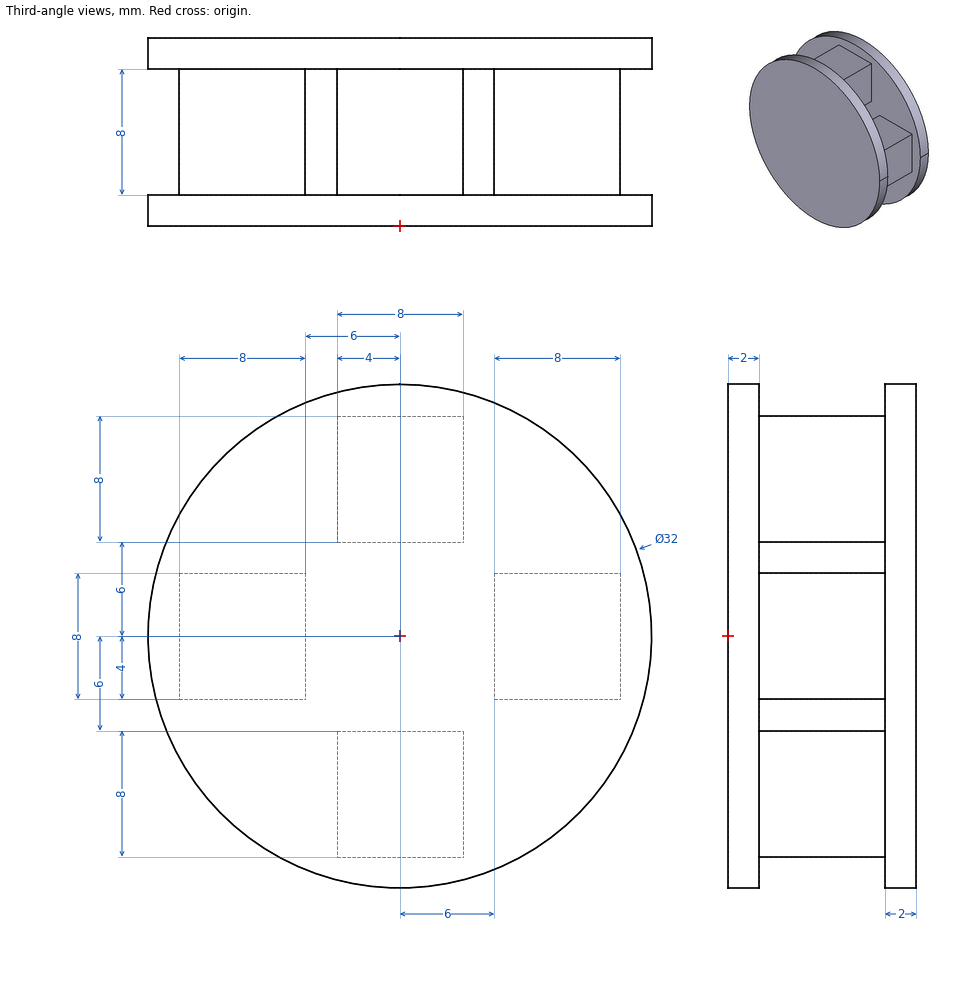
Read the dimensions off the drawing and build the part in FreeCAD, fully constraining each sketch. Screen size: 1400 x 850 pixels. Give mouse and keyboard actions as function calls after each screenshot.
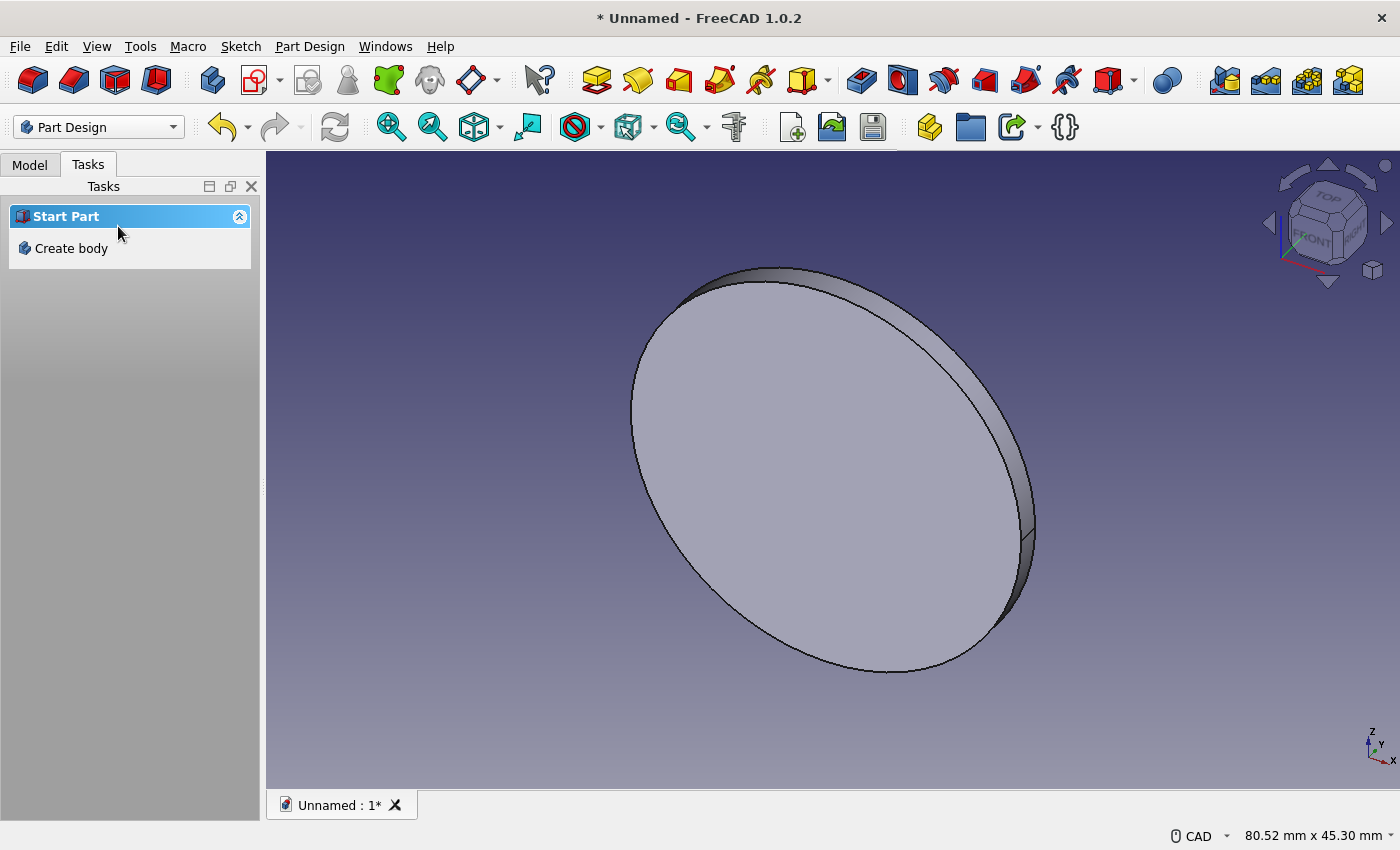
key(4)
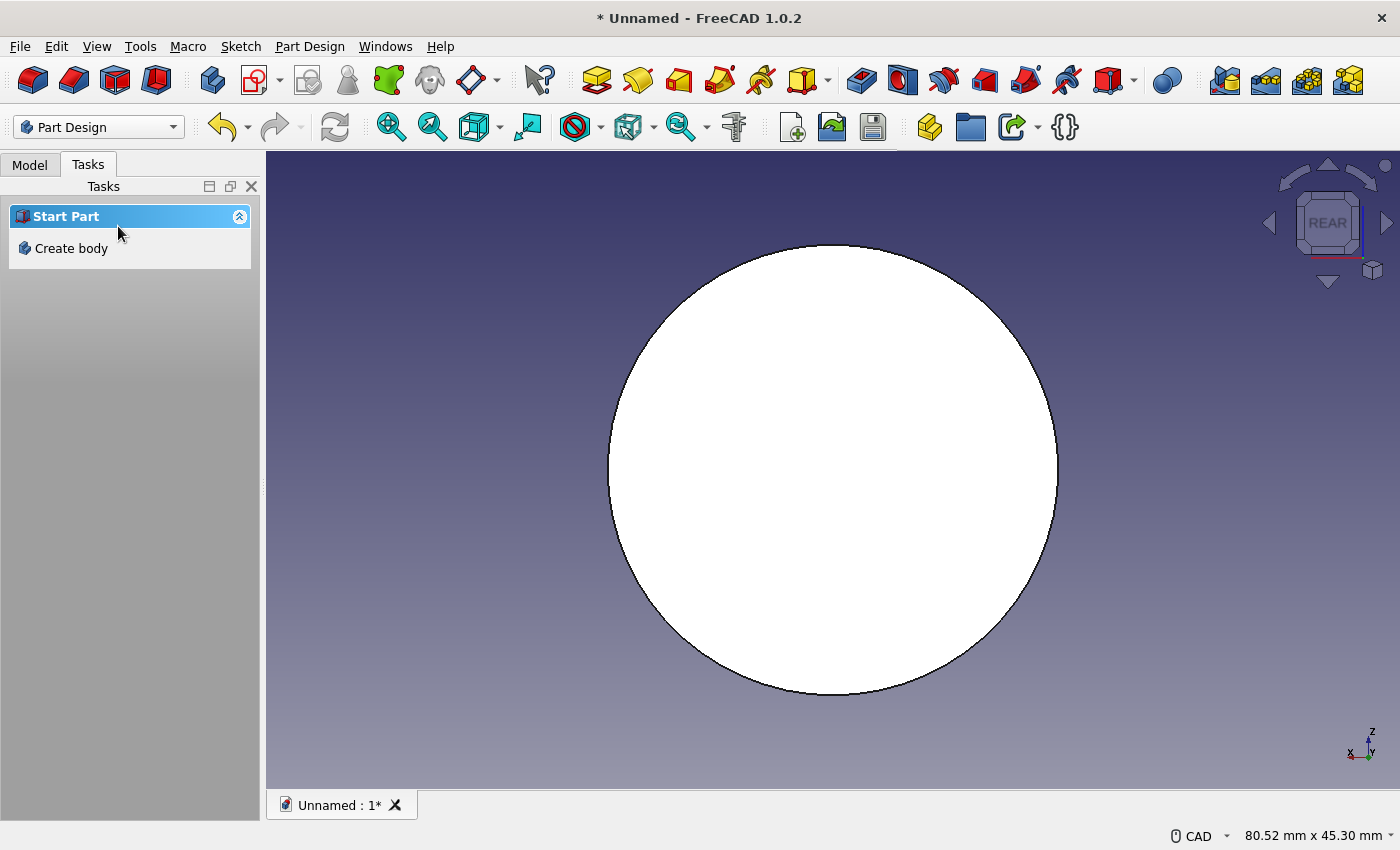
click(833, 469)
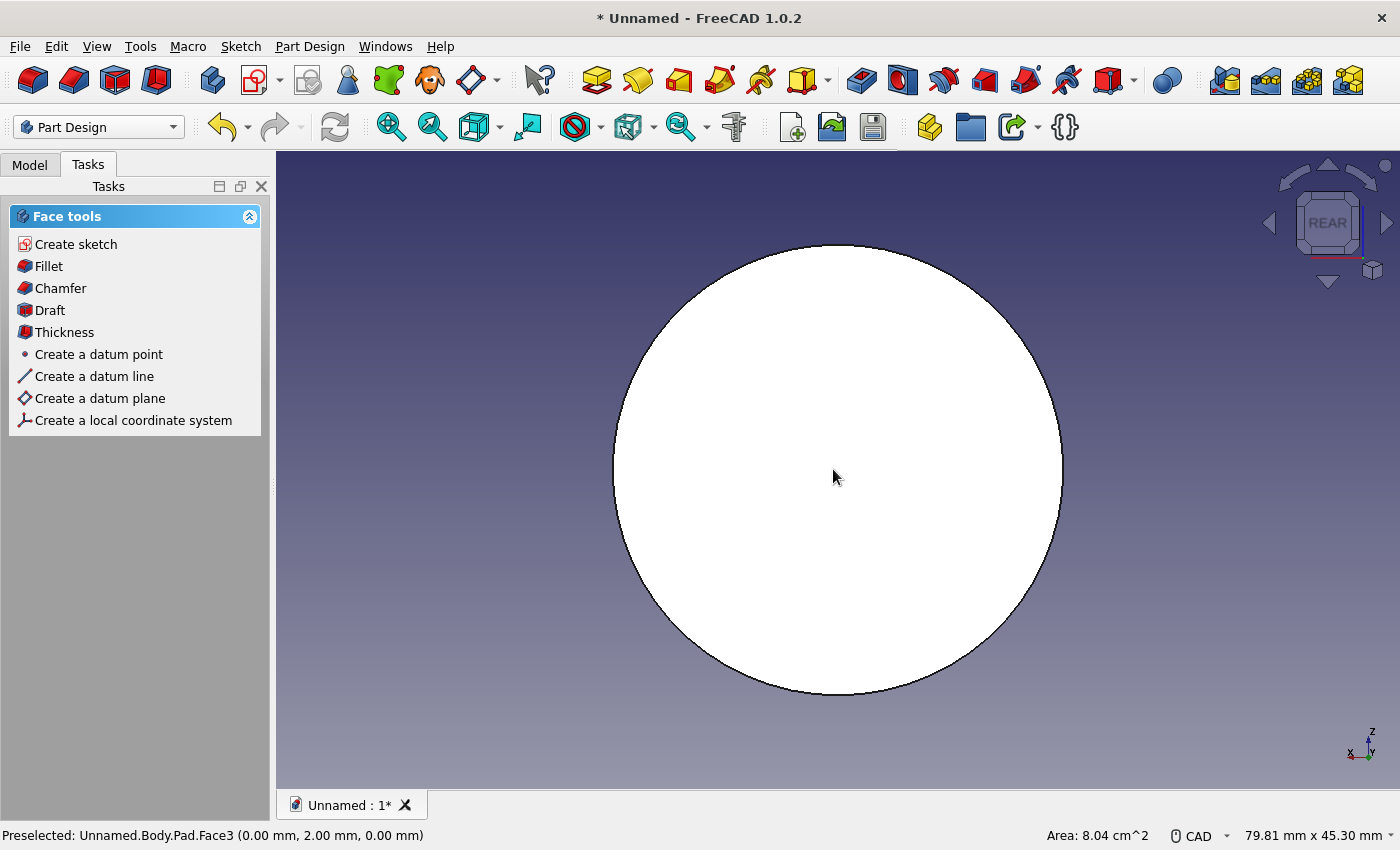
click(254, 80)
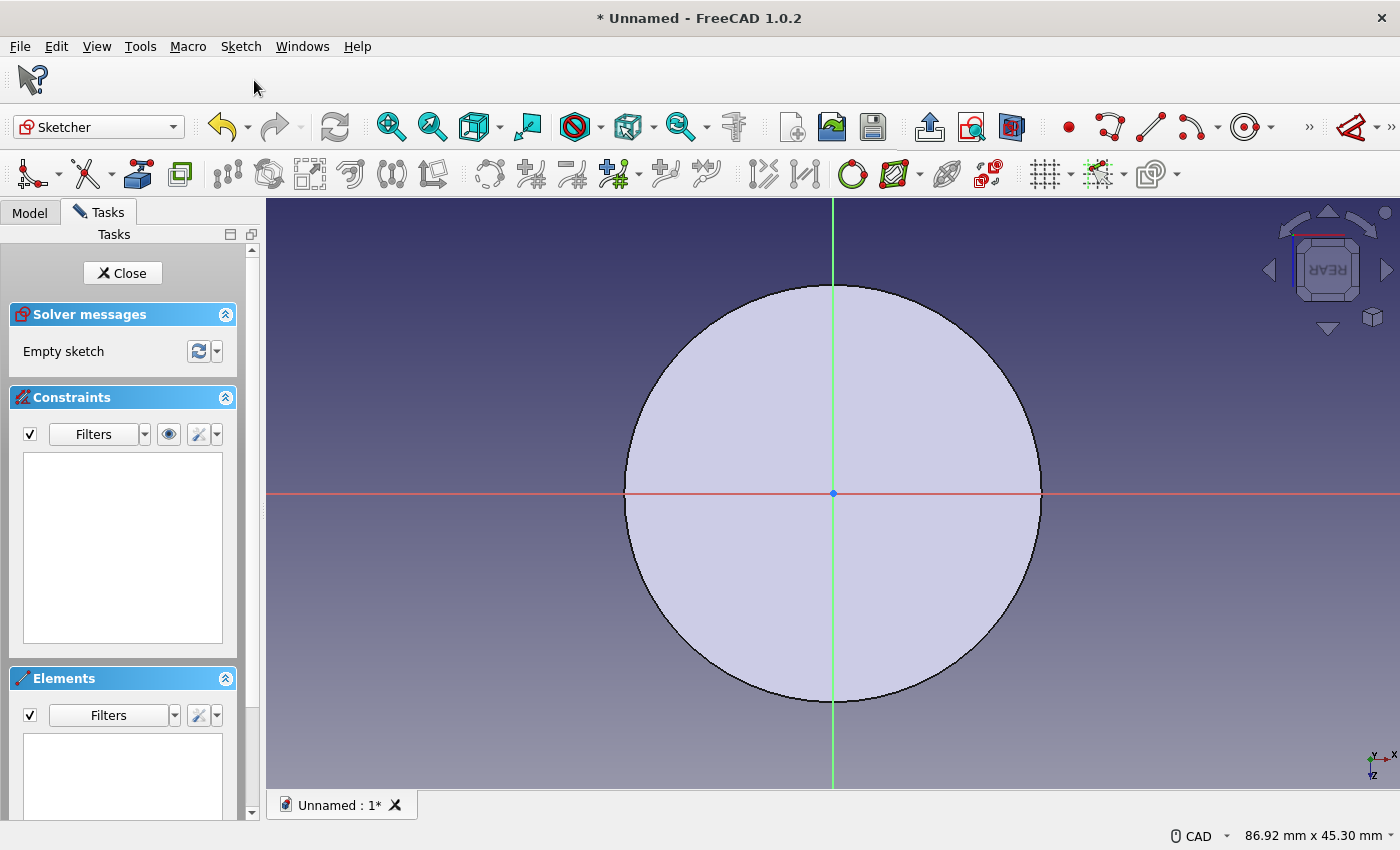
key(g)
key(r)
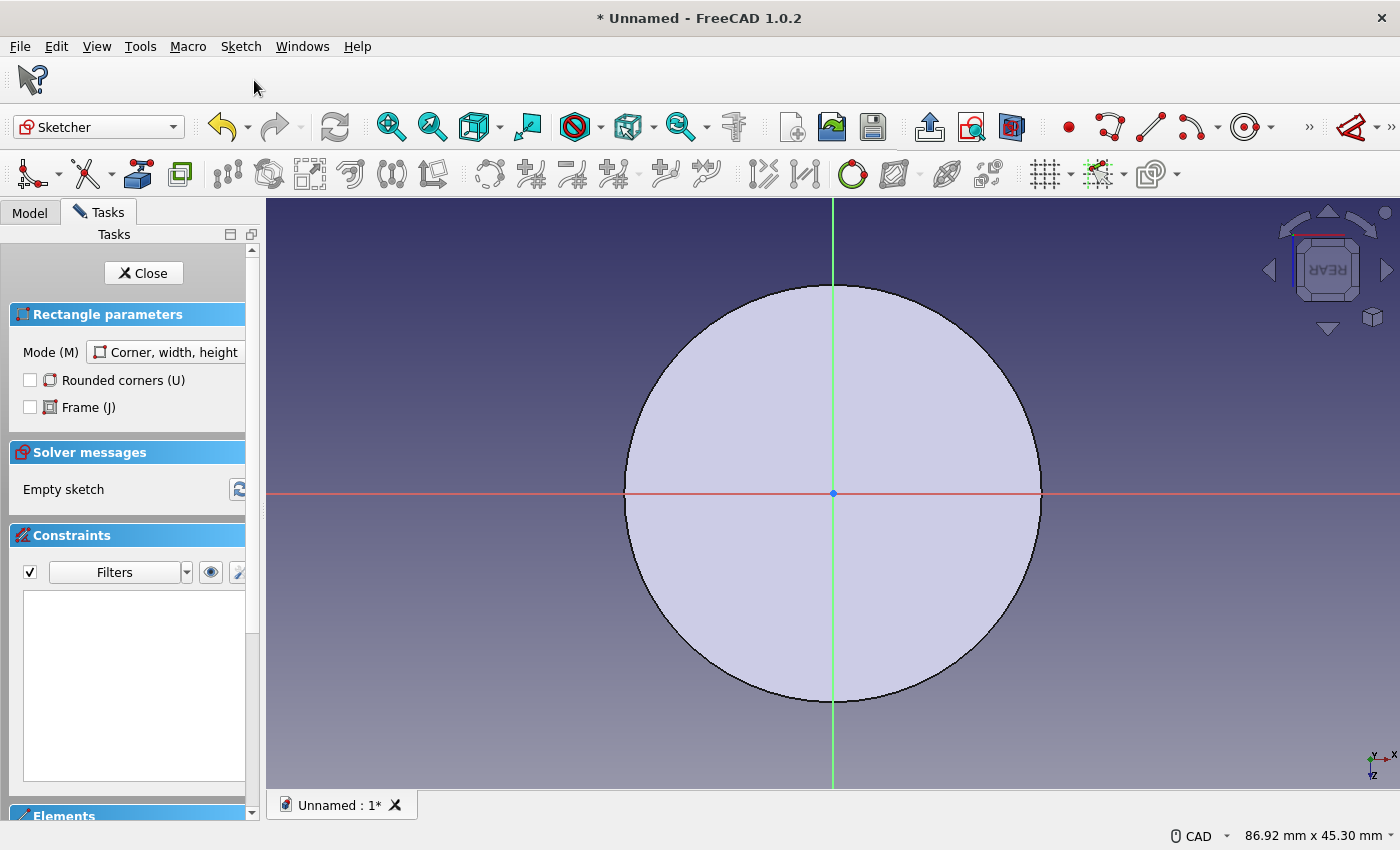
click(650, 441)
click(755, 546)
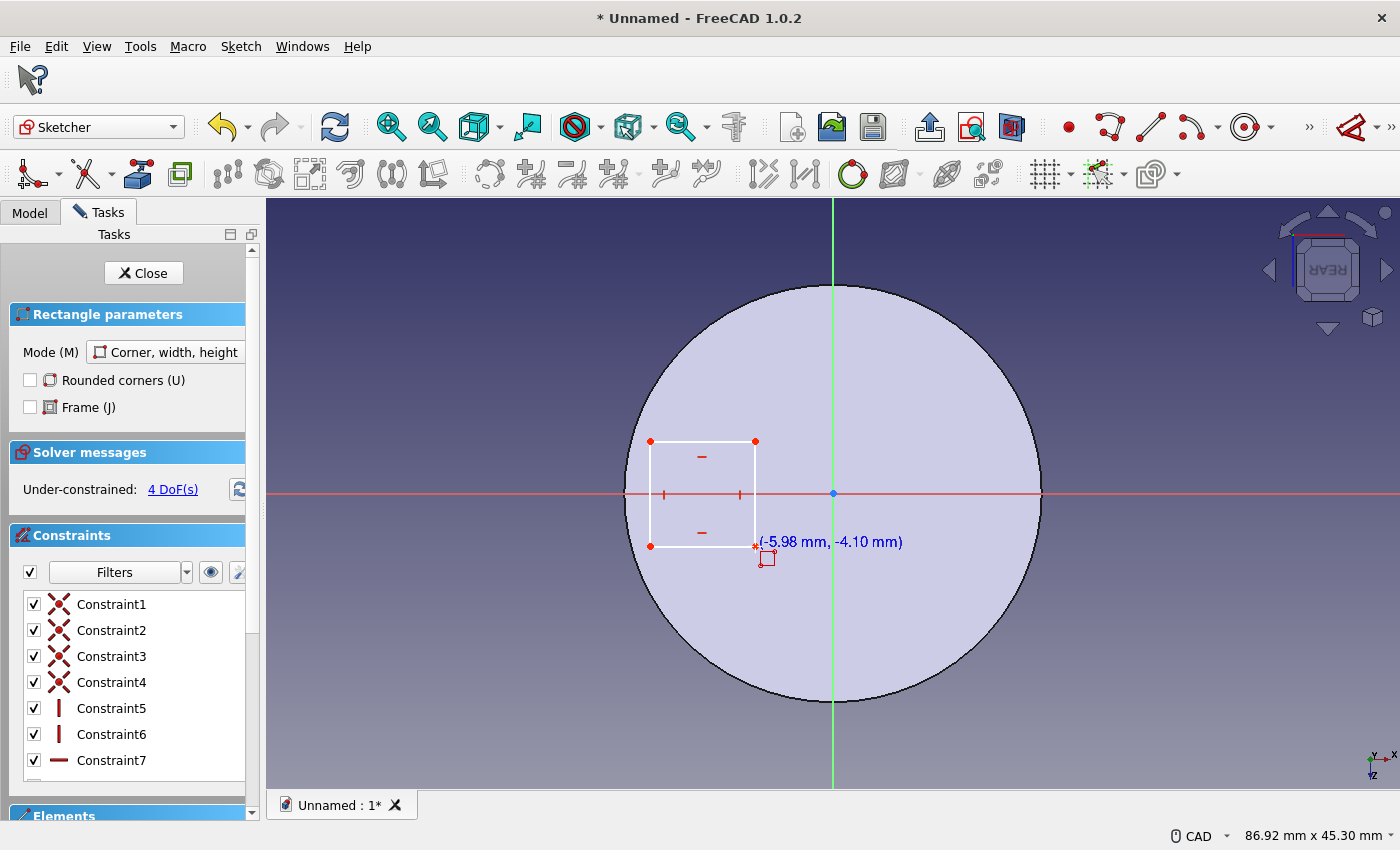
click(781, 572)
click(885, 676)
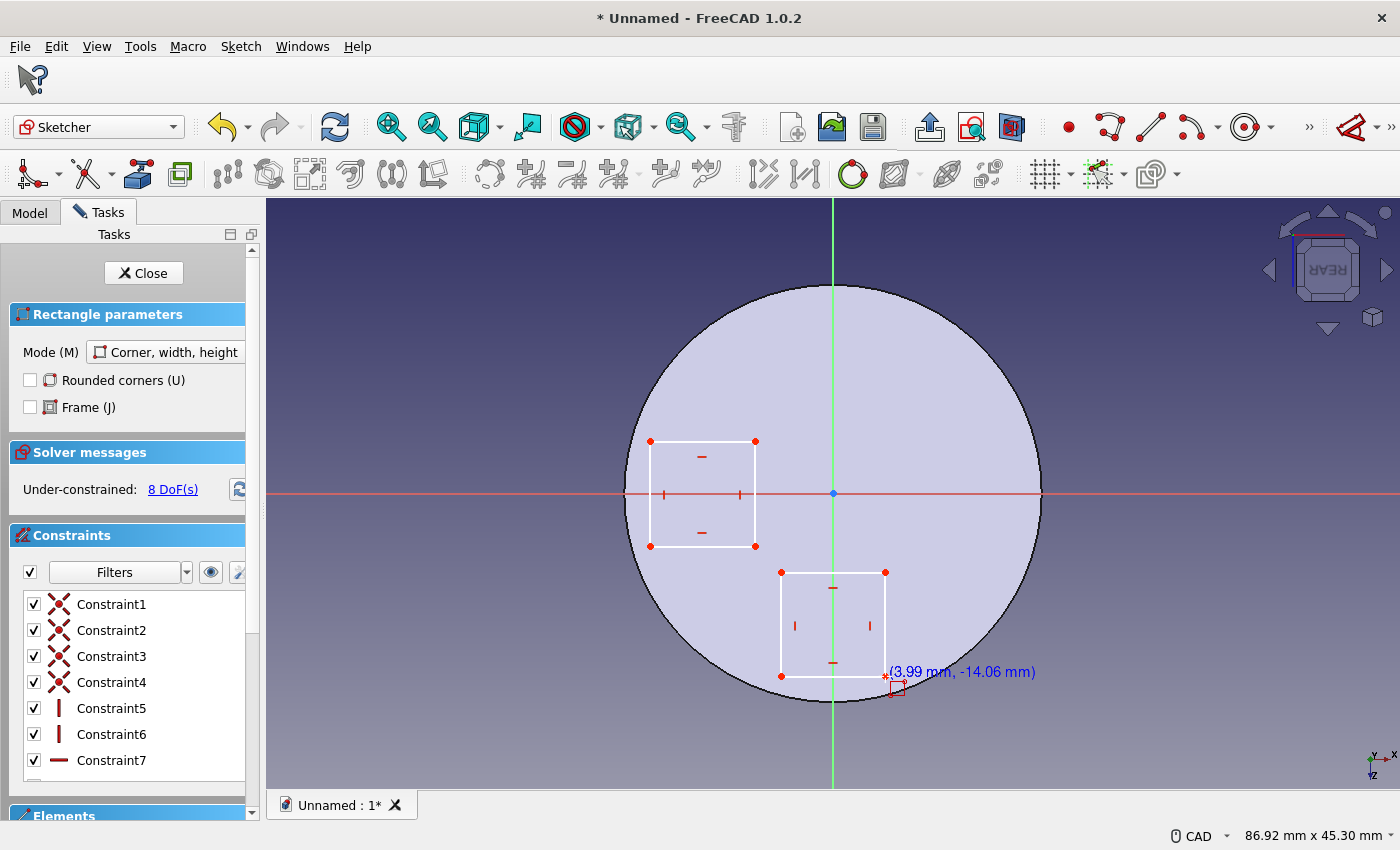
click(781, 311)
click(885, 415)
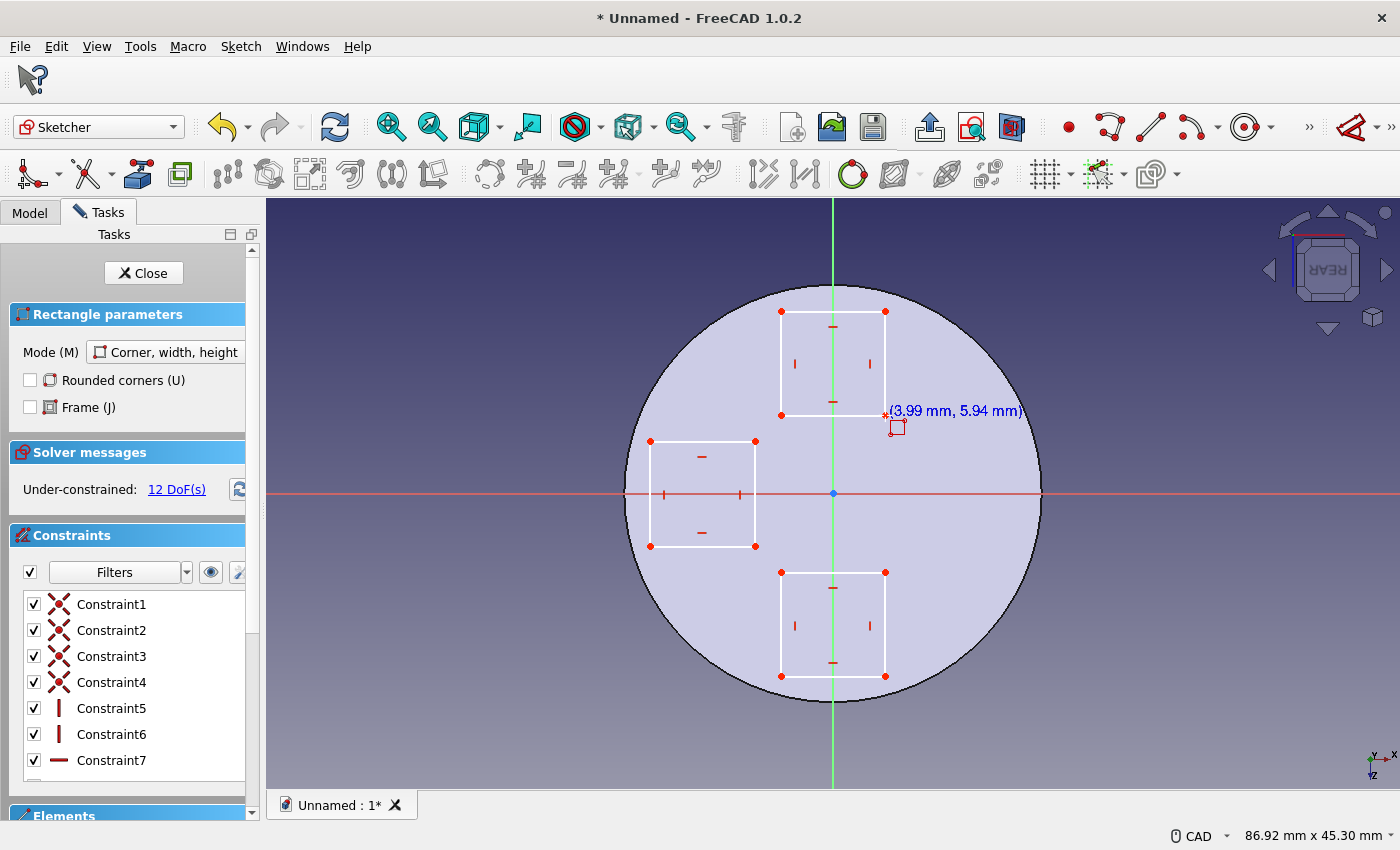
click(911, 441)
click(1016, 546)
key(Escape)